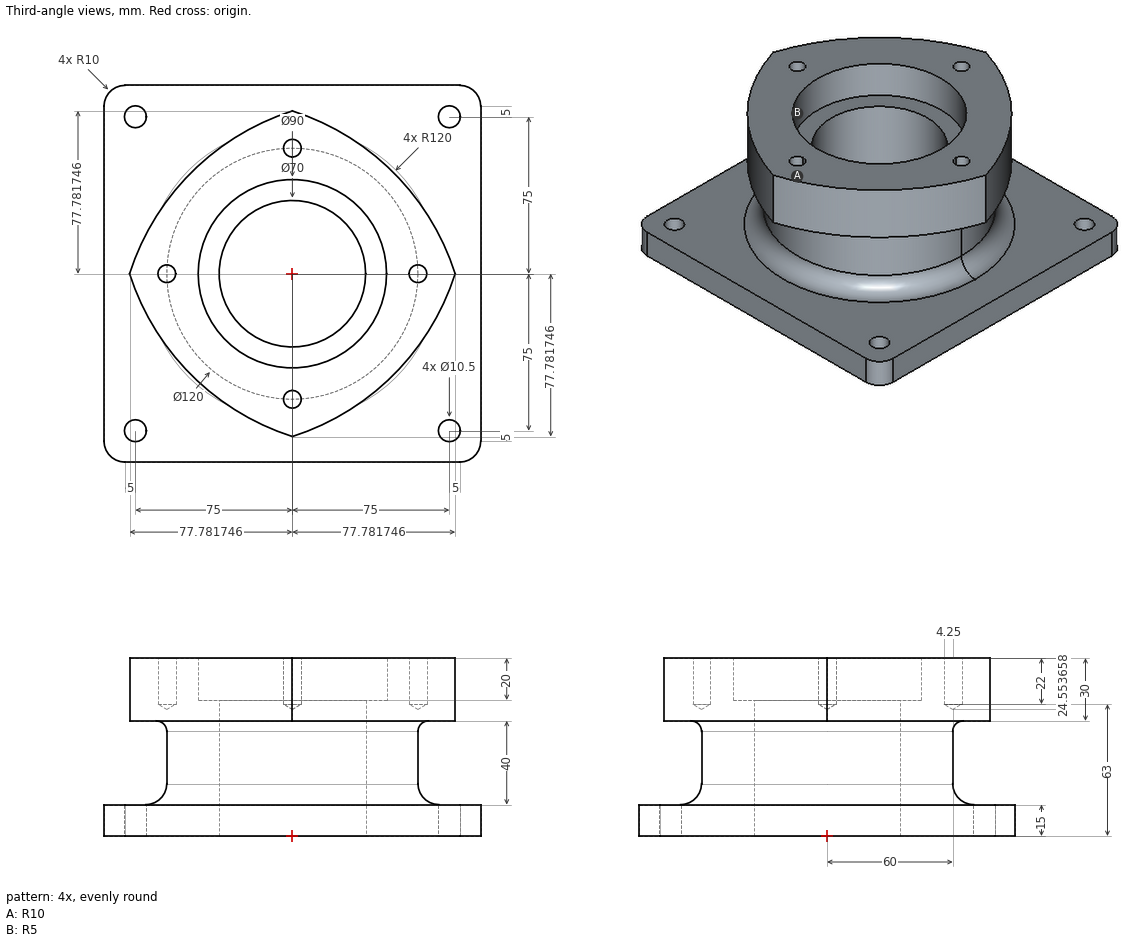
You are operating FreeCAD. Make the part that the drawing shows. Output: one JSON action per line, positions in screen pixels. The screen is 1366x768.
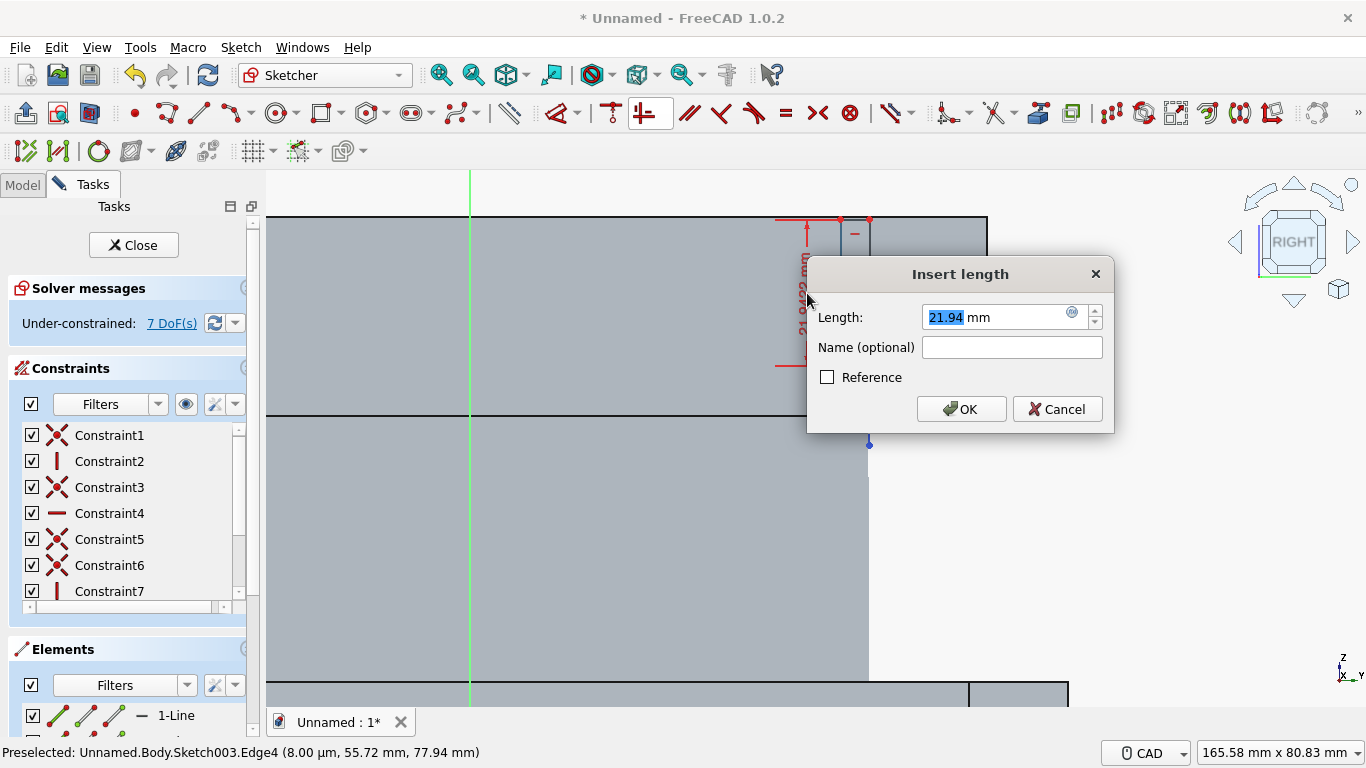
{"action": "type", "text": "22"}
{"action": "key", "text": "Return"}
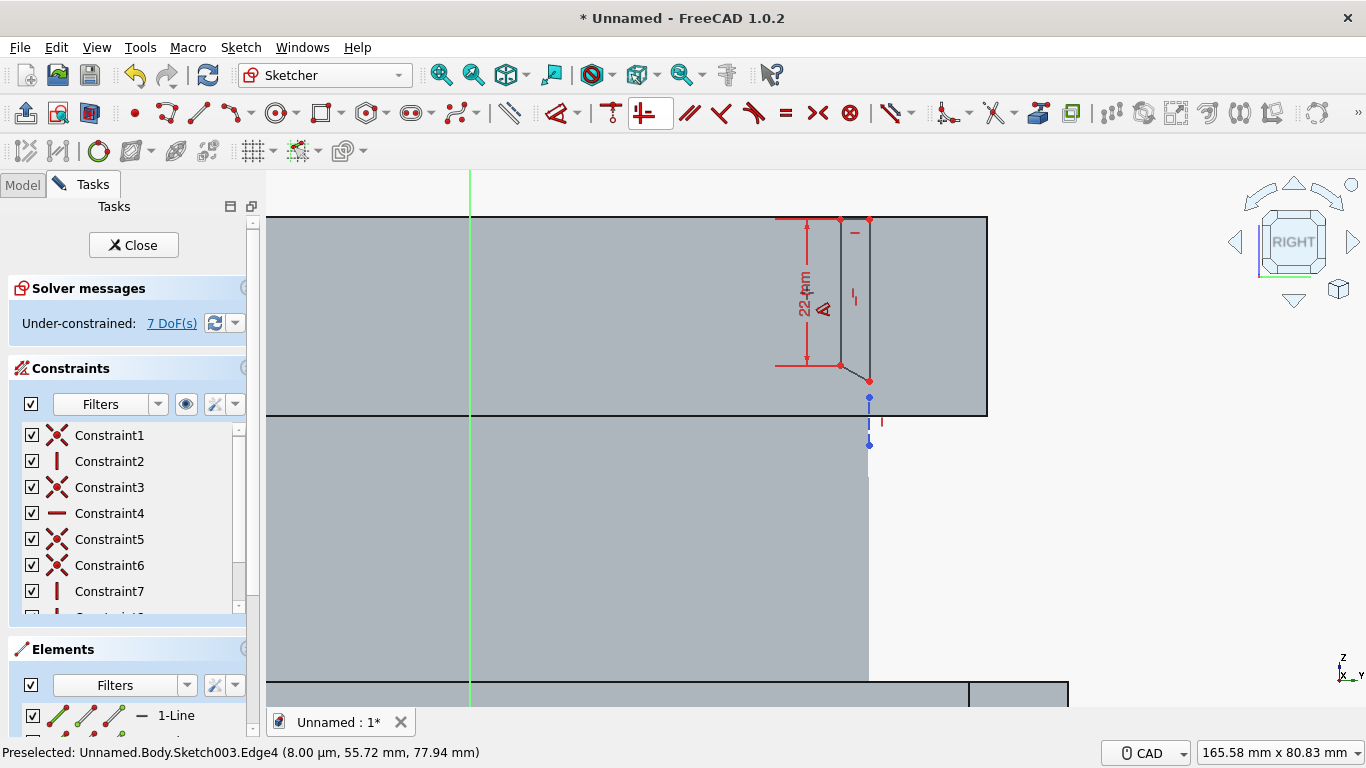
{"action": "left_click", "coordinate": [841, 366]}
{"action": "left_click", "coordinate": [436, 522]}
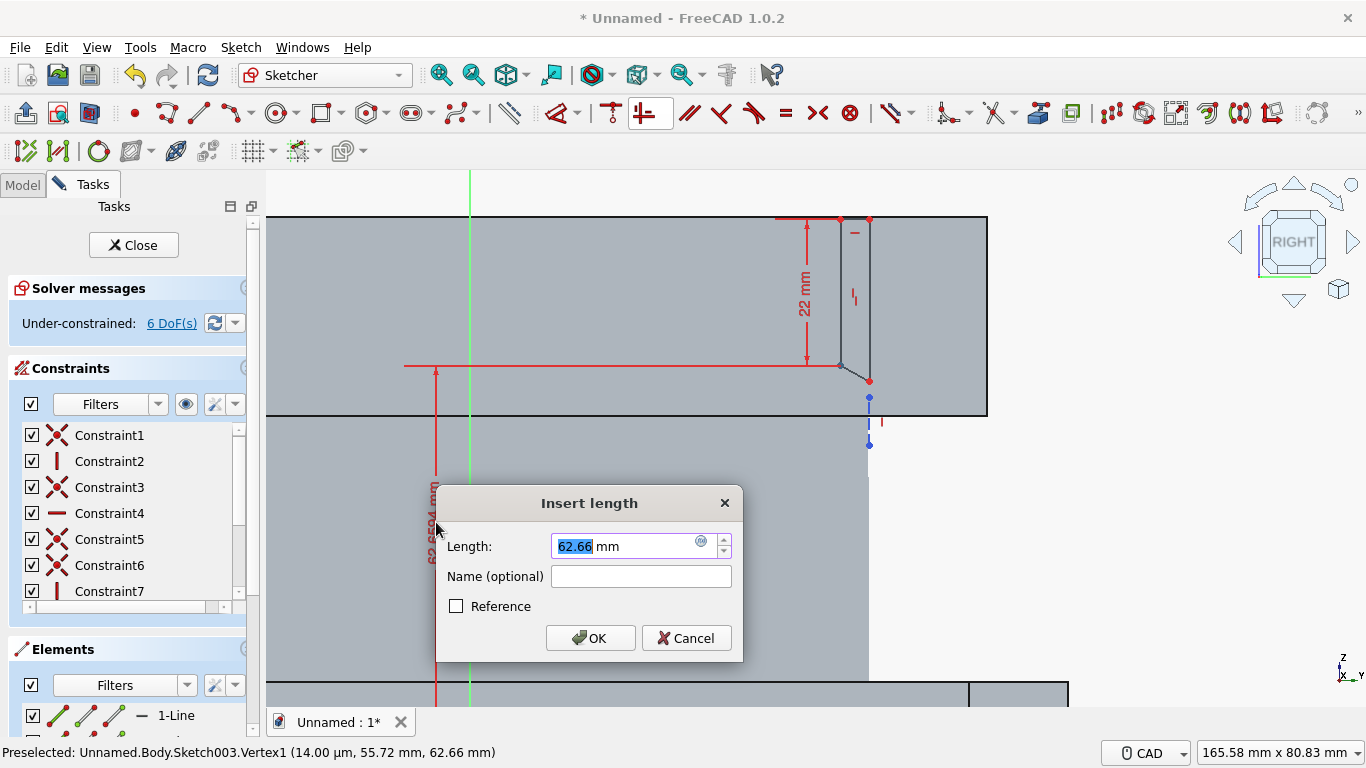
{"action": "type", "text": "63"}
{"action": "key", "text": "Return"}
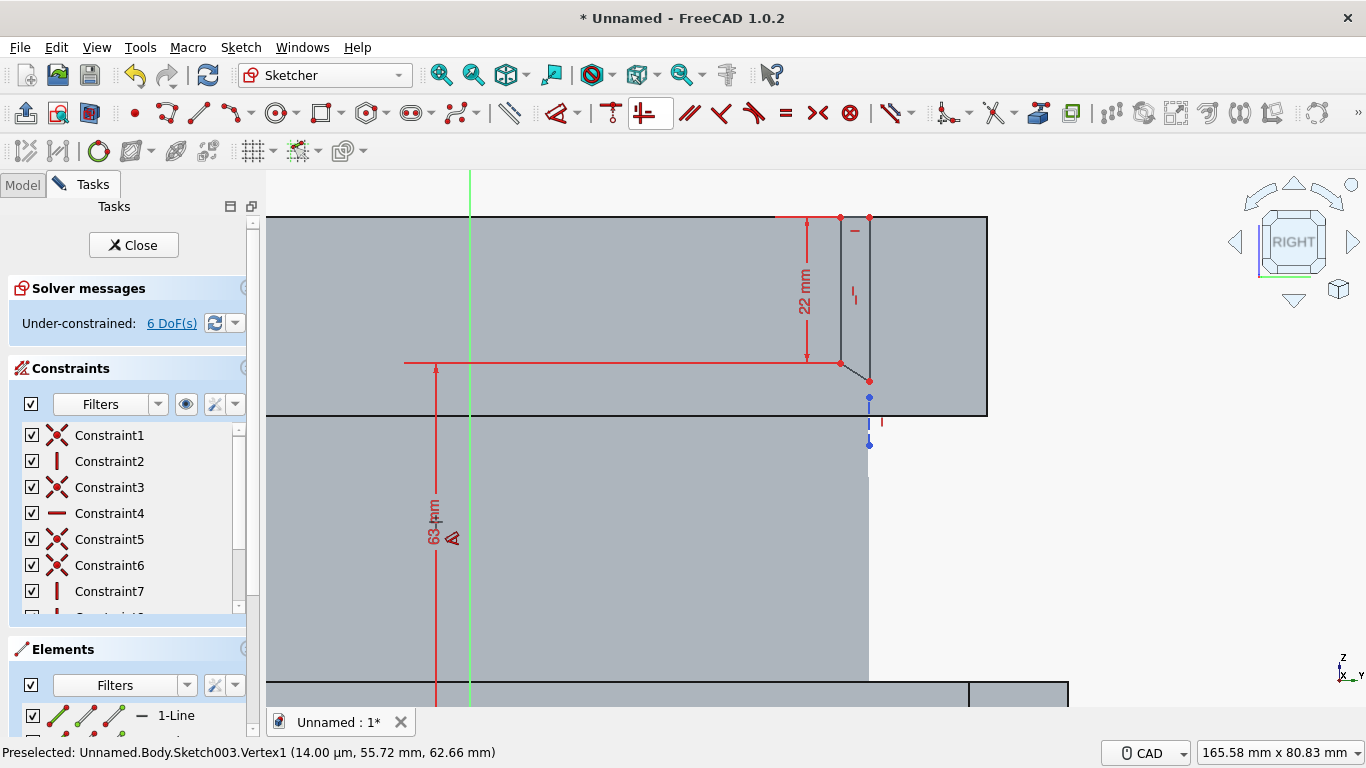
{"action": "left_click", "coordinate": [870, 382]}
{"action": "left_click", "coordinate": [670, 348]}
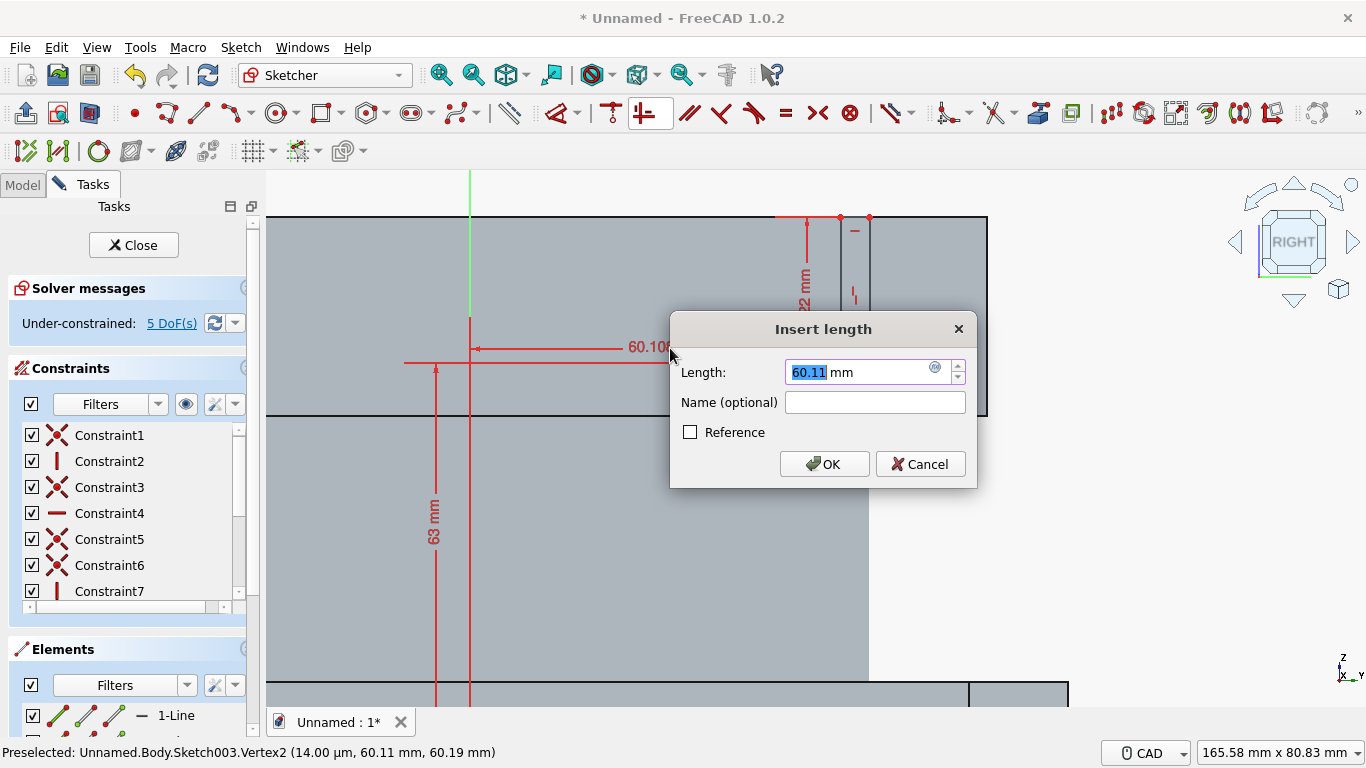
{"action": "type", "text": "60"}
{"action": "key", "text": "Return"}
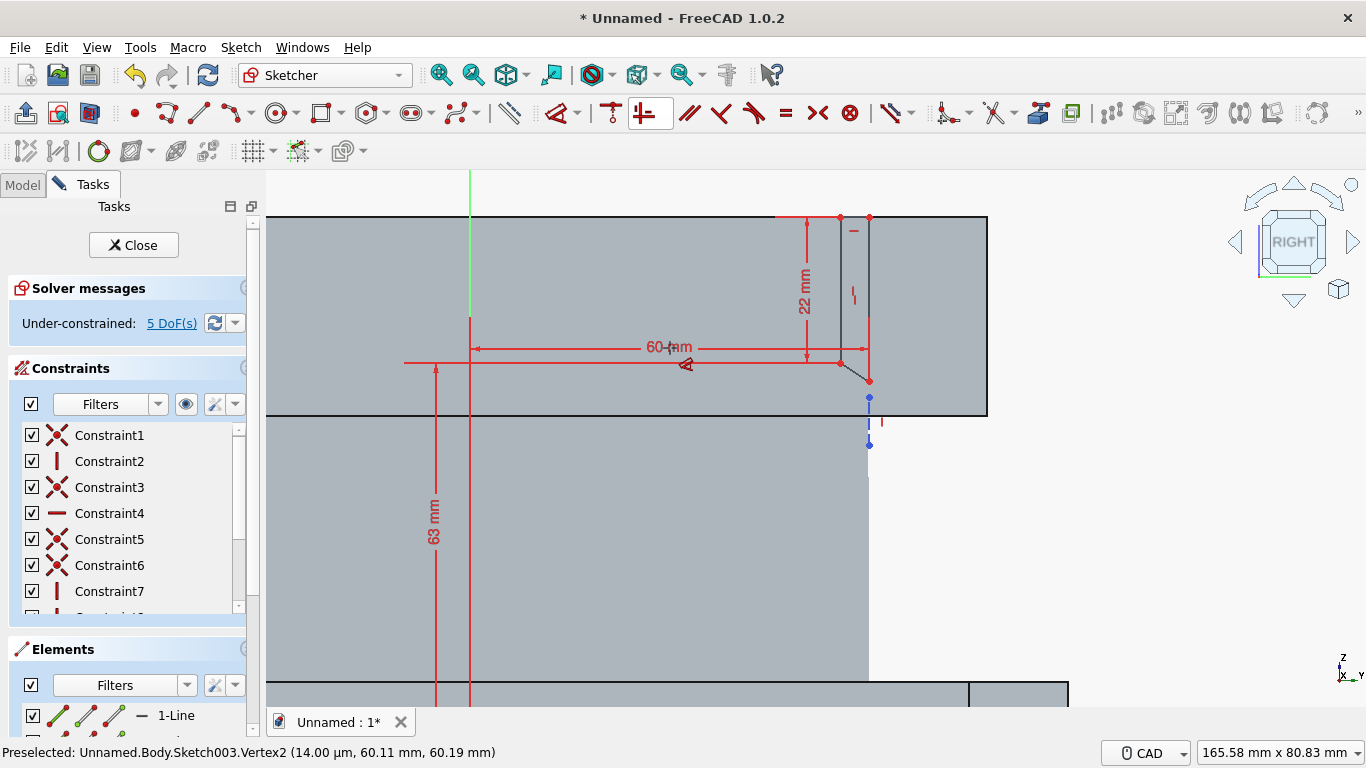
{"action": "left_click", "coordinate": [869, 398]}
{"action": "left_click", "coordinate": [578, 364]}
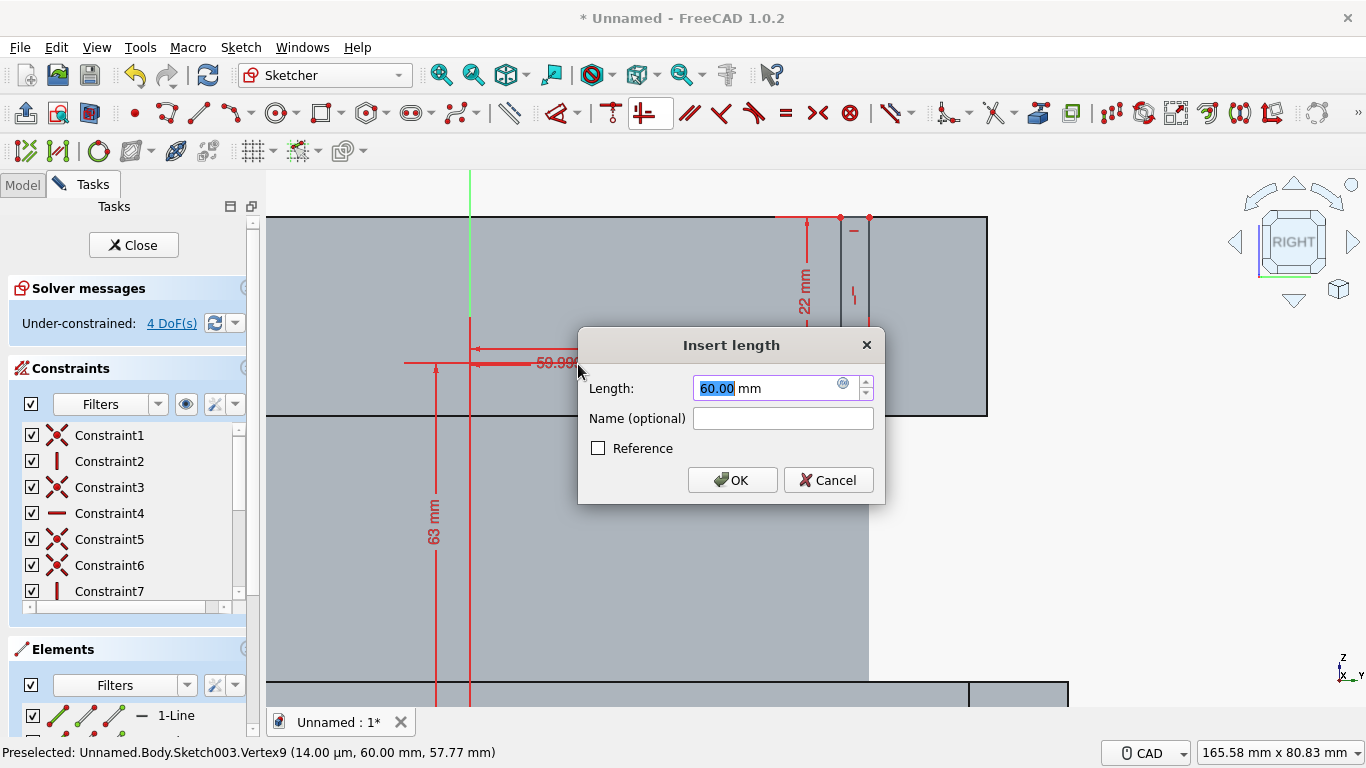
{"action": "type", "text": "60"}
{"action": "key", "text": "Return"}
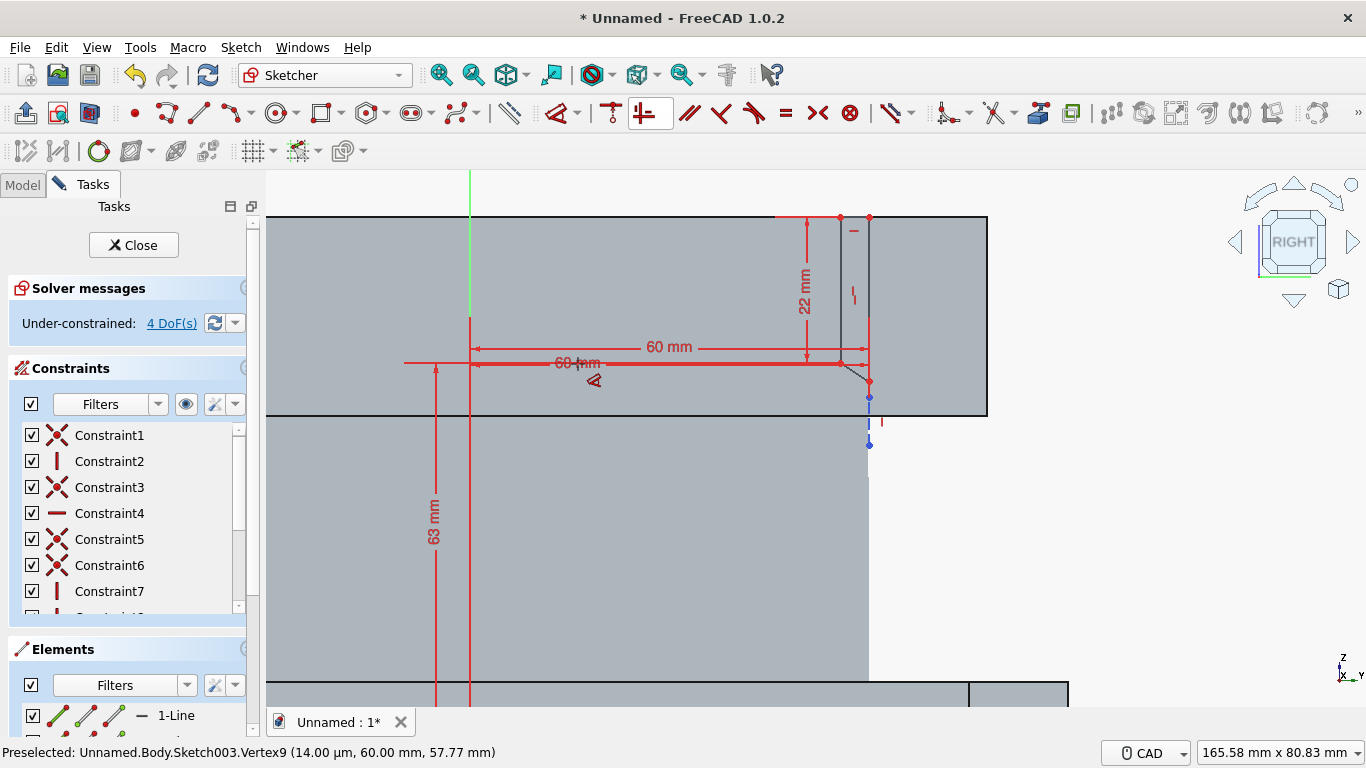
{"action": "scroll", "coordinate": [858, 217], "scroll_direction": "up", "scroll_amount": 2}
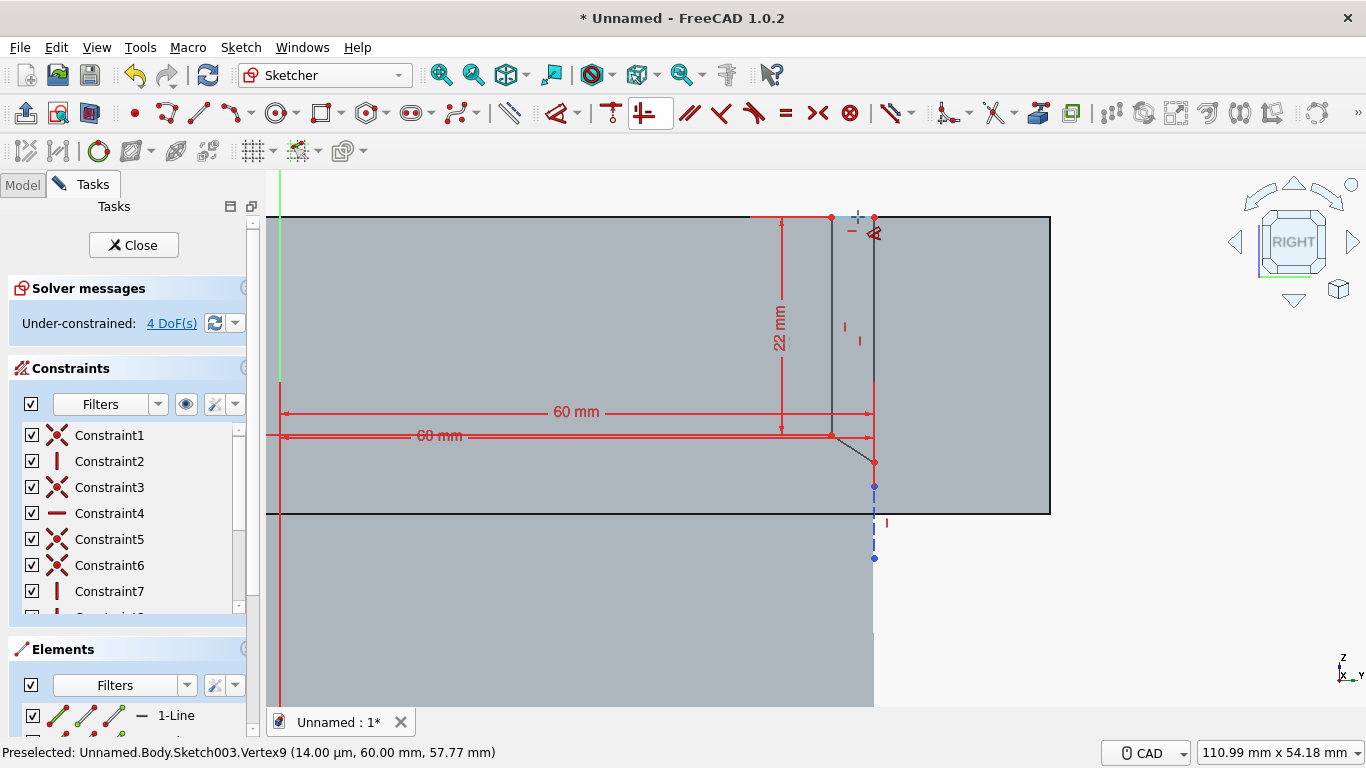
{"action": "left_click", "coordinate": [857, 217]}
{"action": "left_click", "coordinate": [853, 251]}